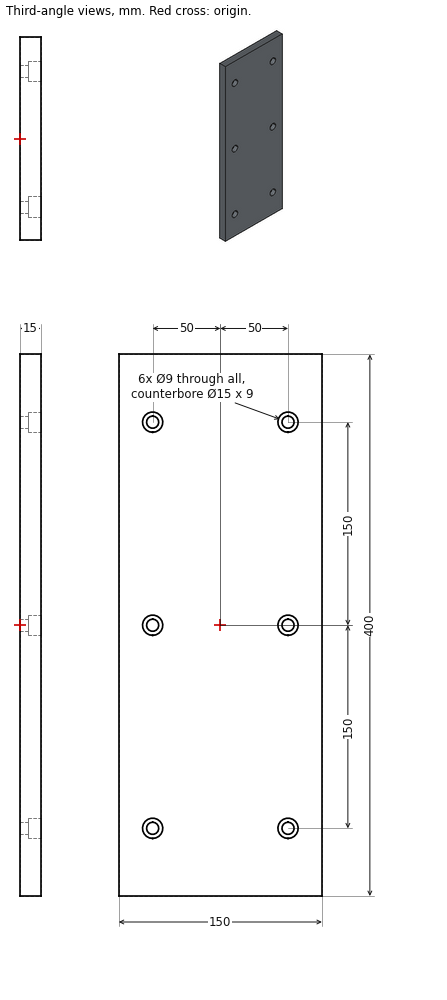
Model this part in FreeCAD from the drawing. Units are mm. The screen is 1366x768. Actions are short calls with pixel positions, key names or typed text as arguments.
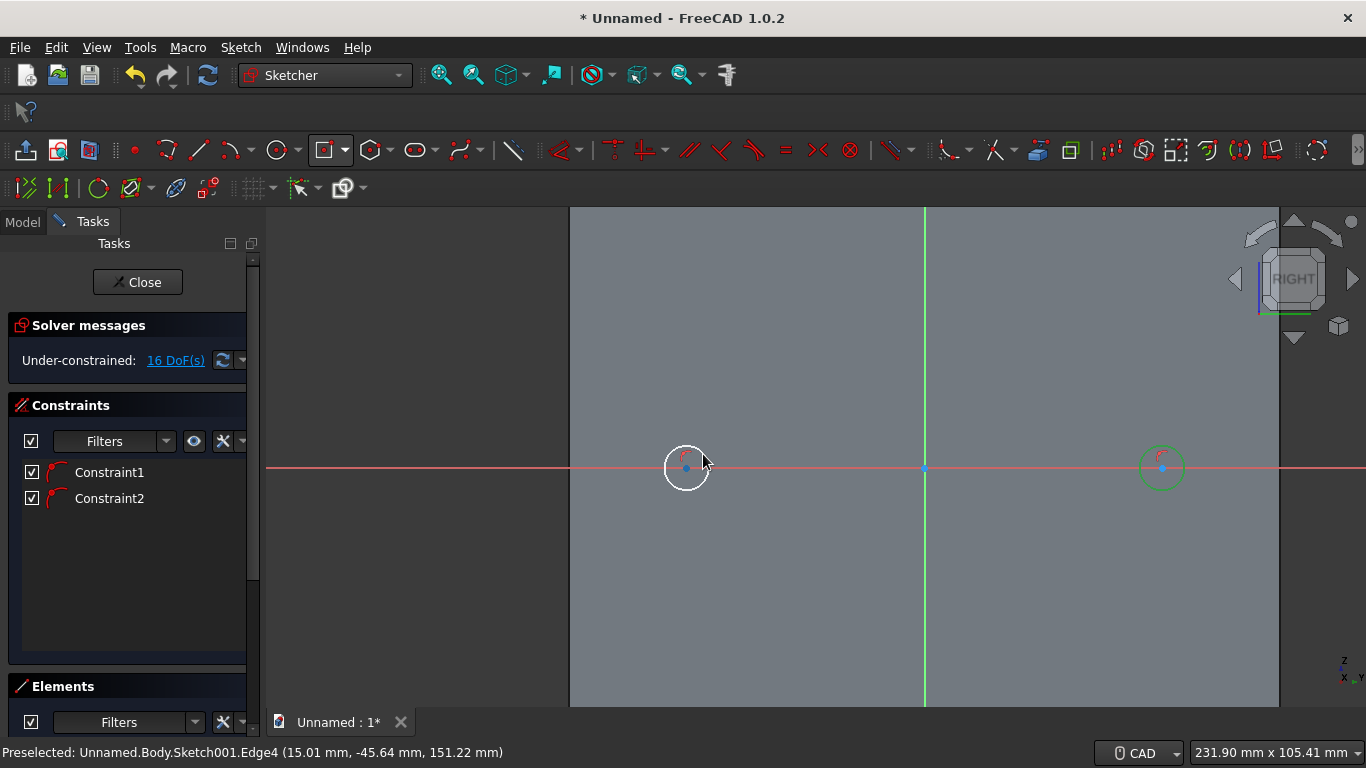
click(702, 452)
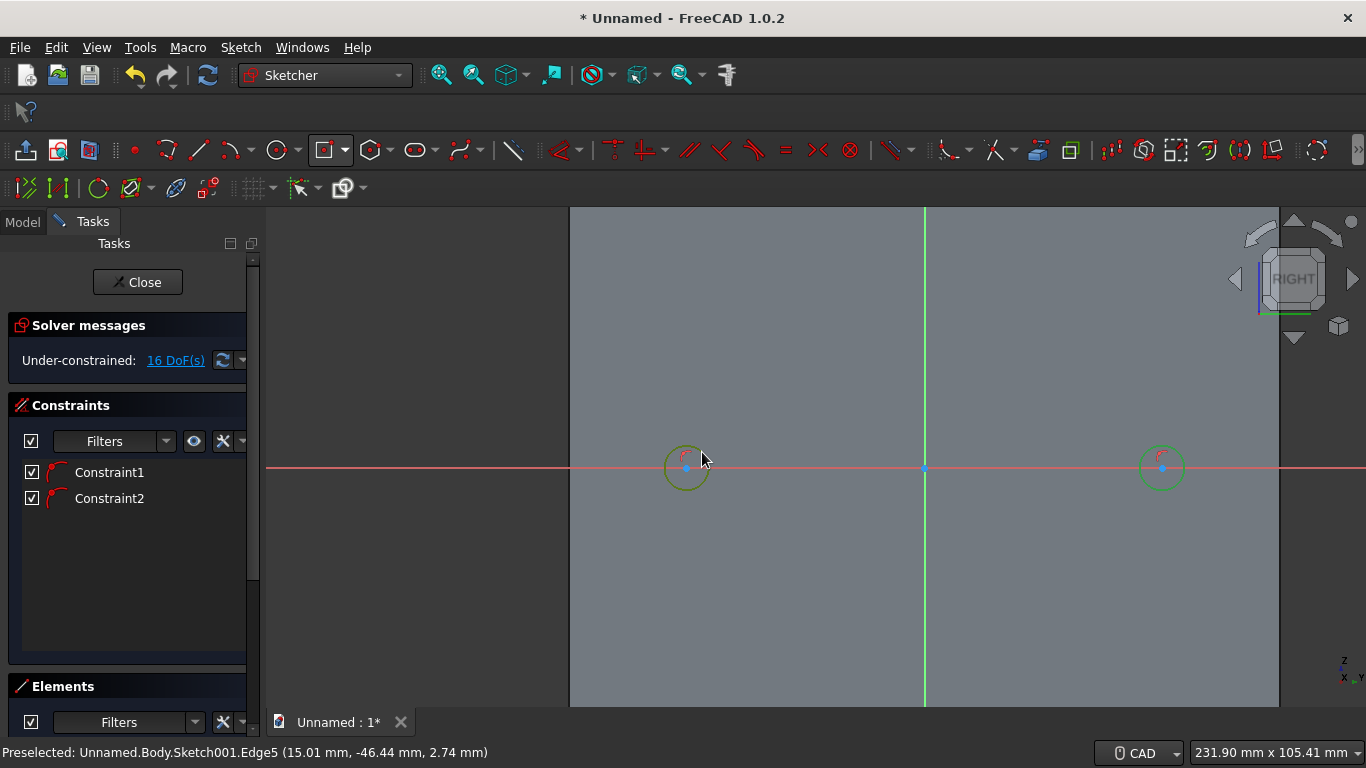
scroll(703, 454, down, 8)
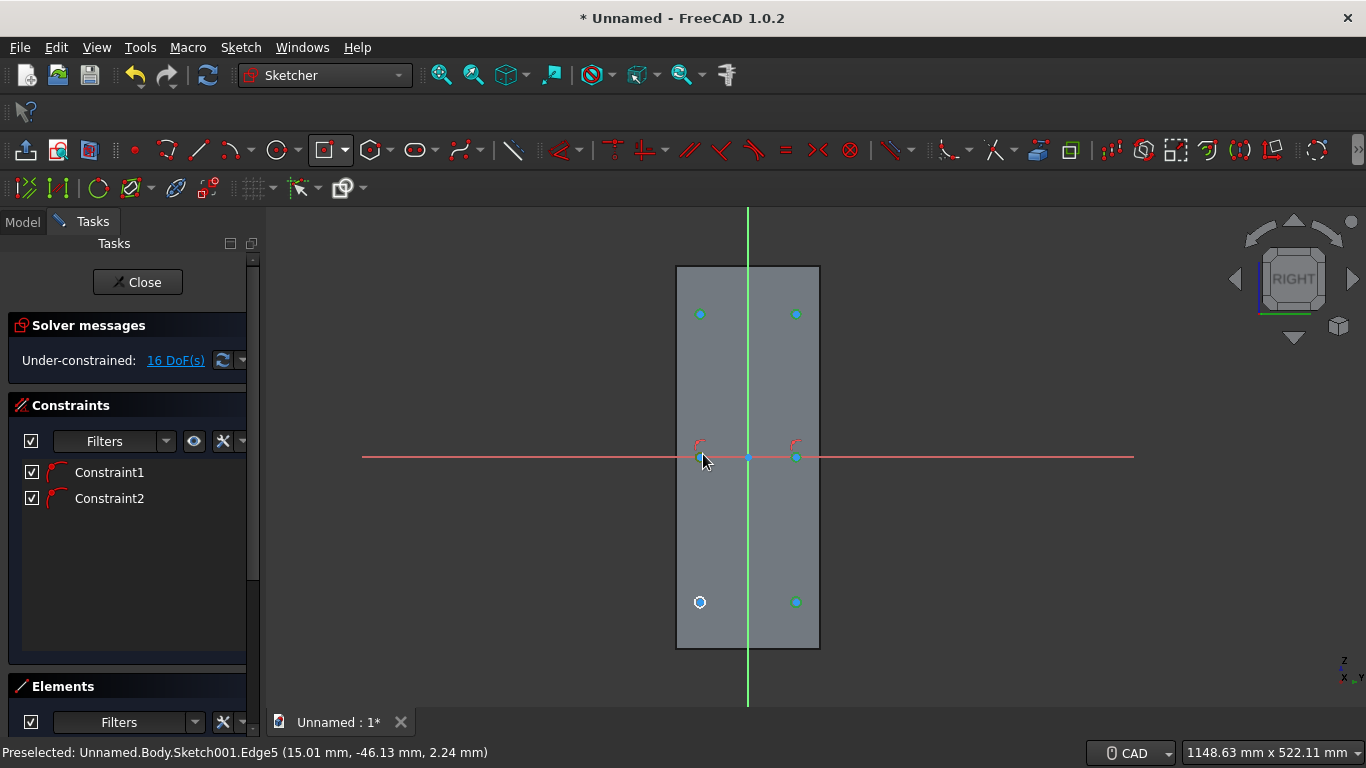
scroll(704, 599, up, 5)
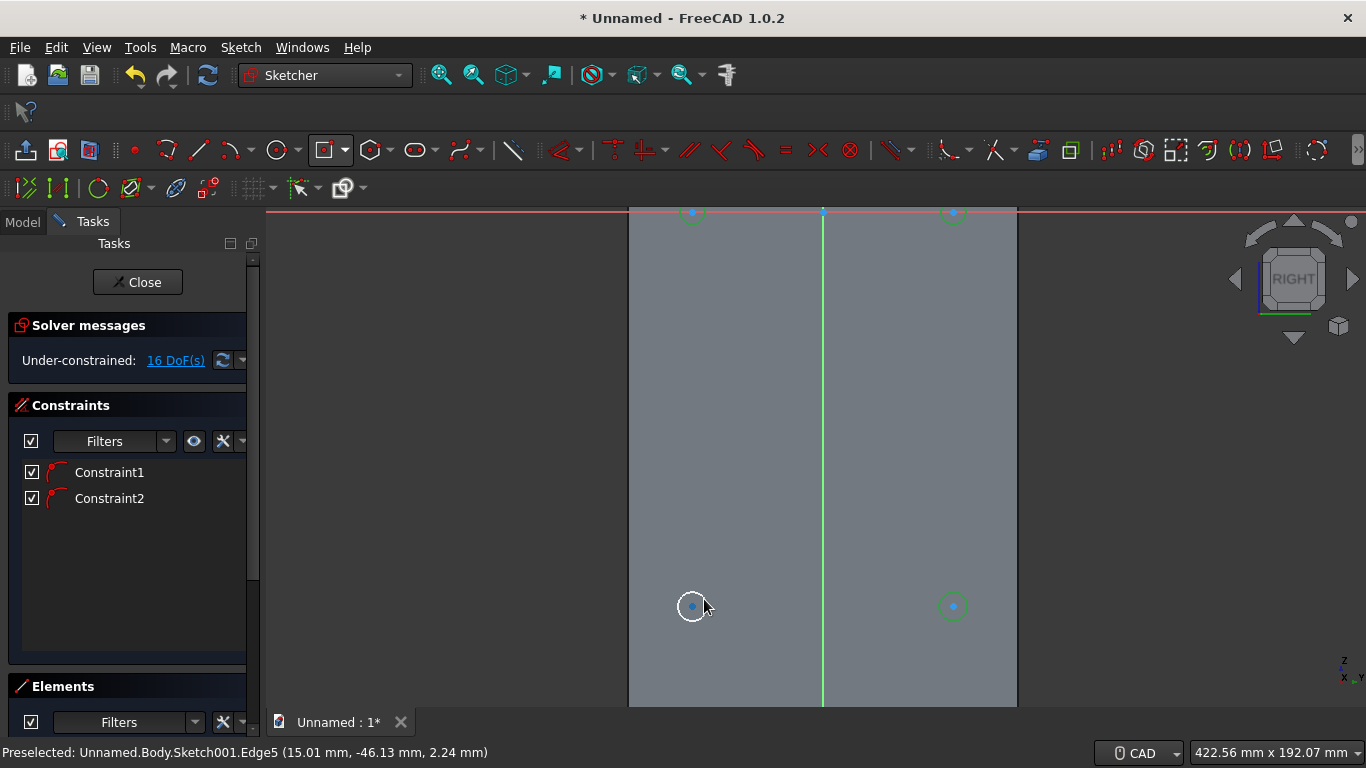
click(703, 596)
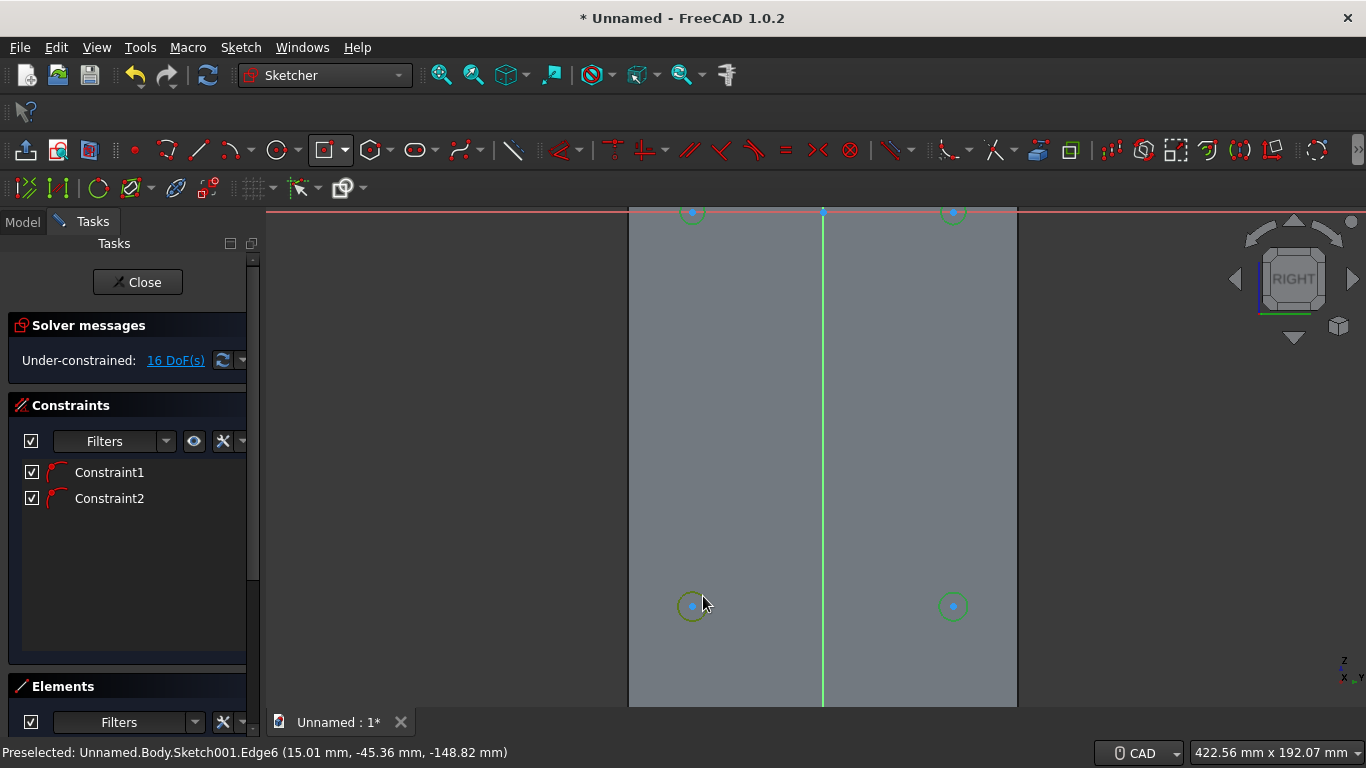
key(e)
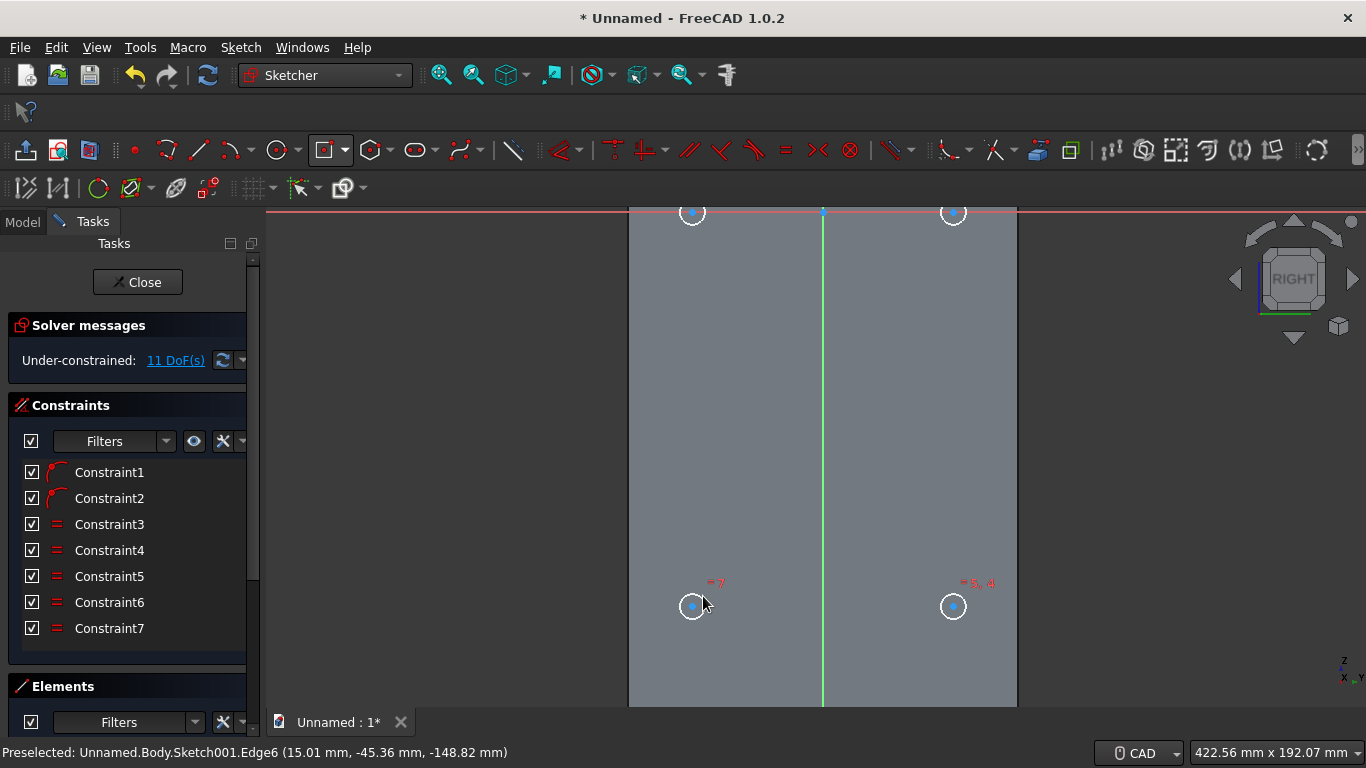
scroll(703, 599, down, 5)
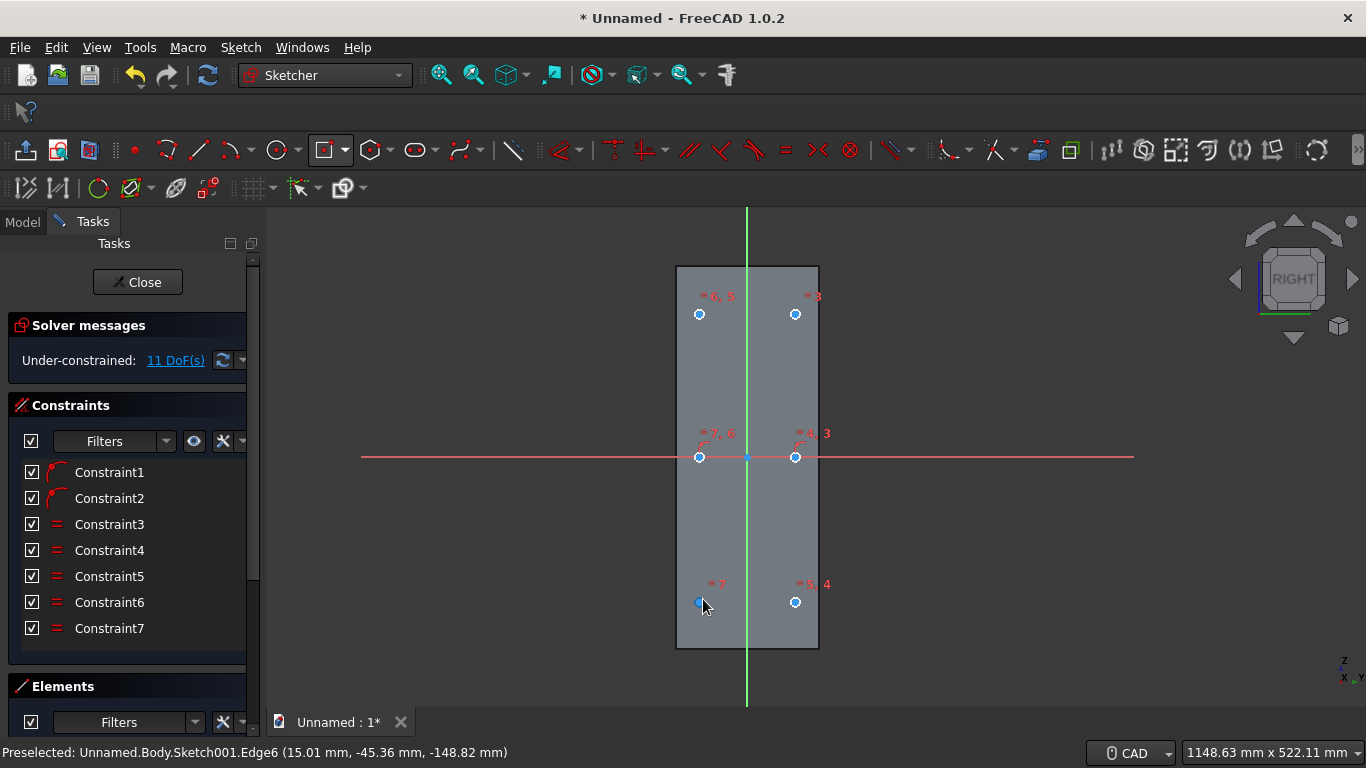
click(795, 314)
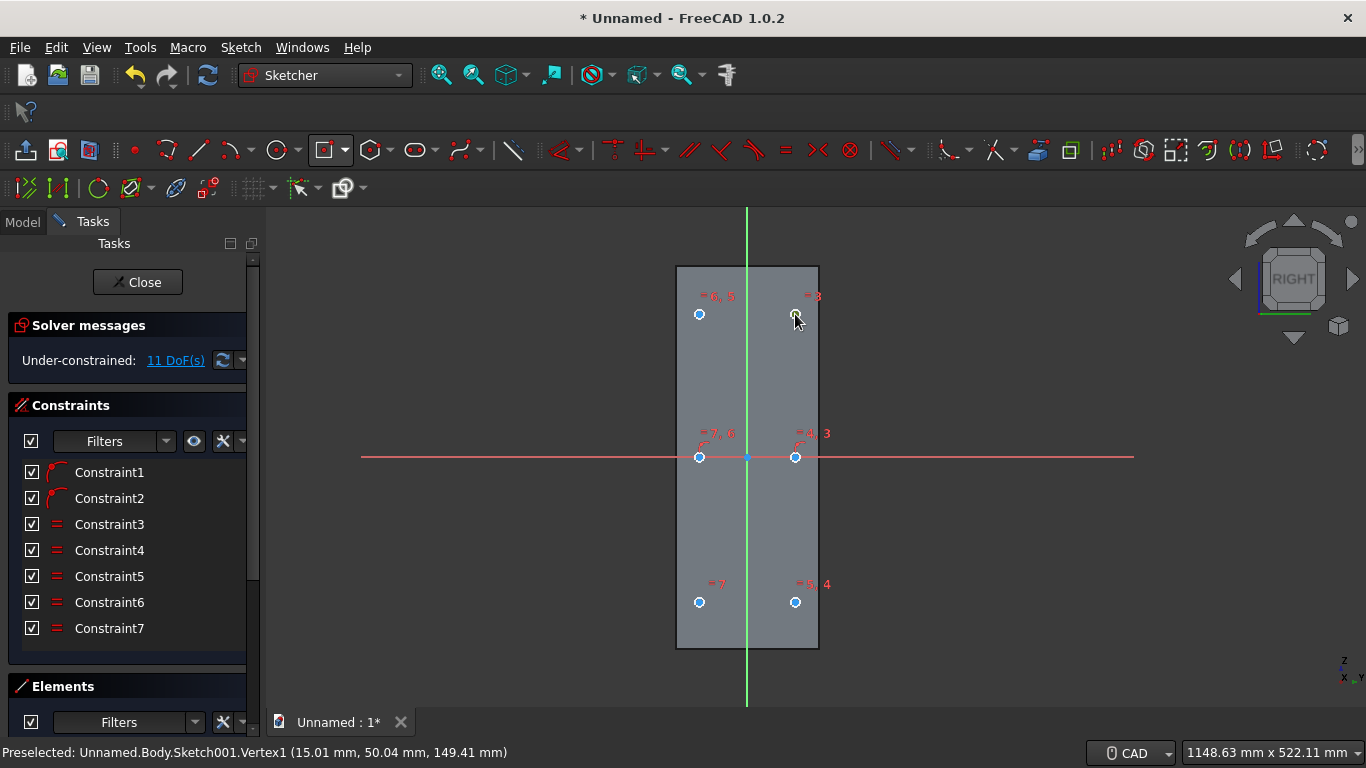
click(795, 457)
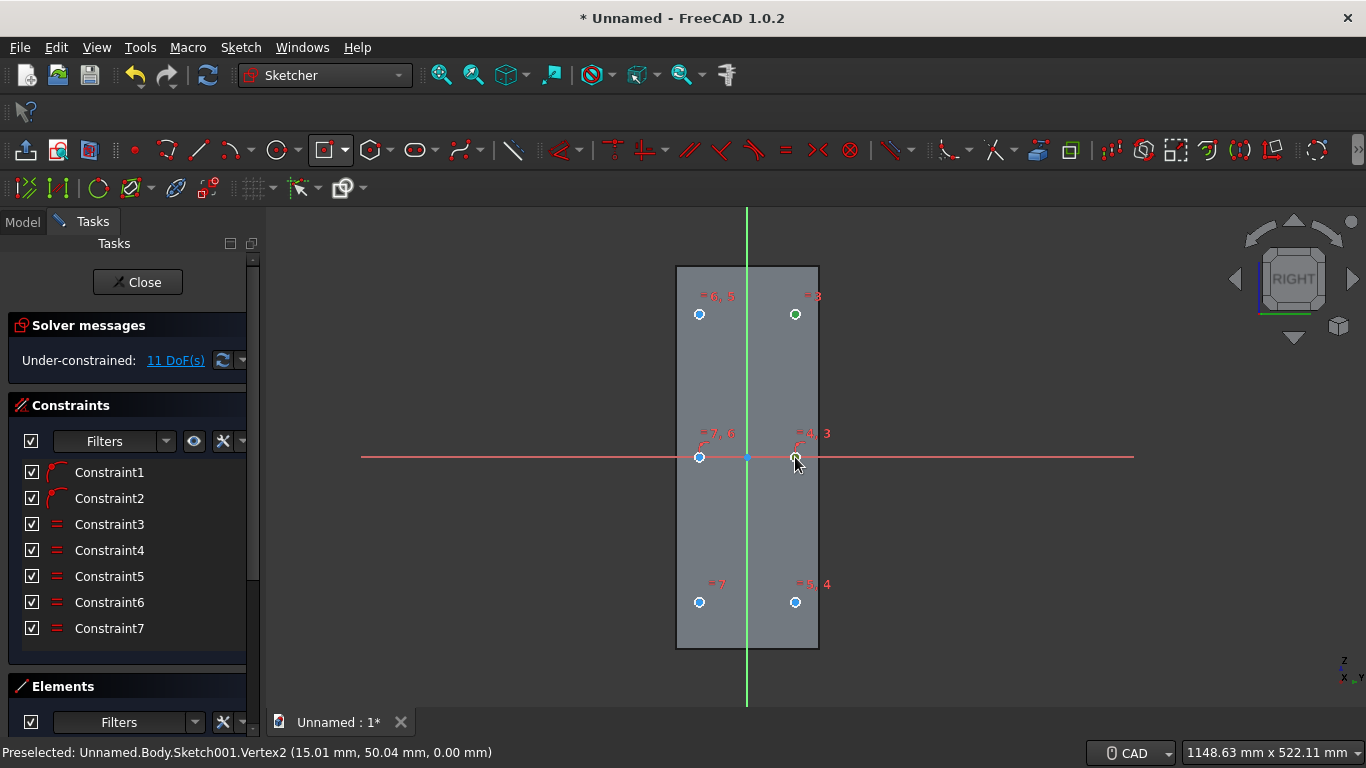
key(v)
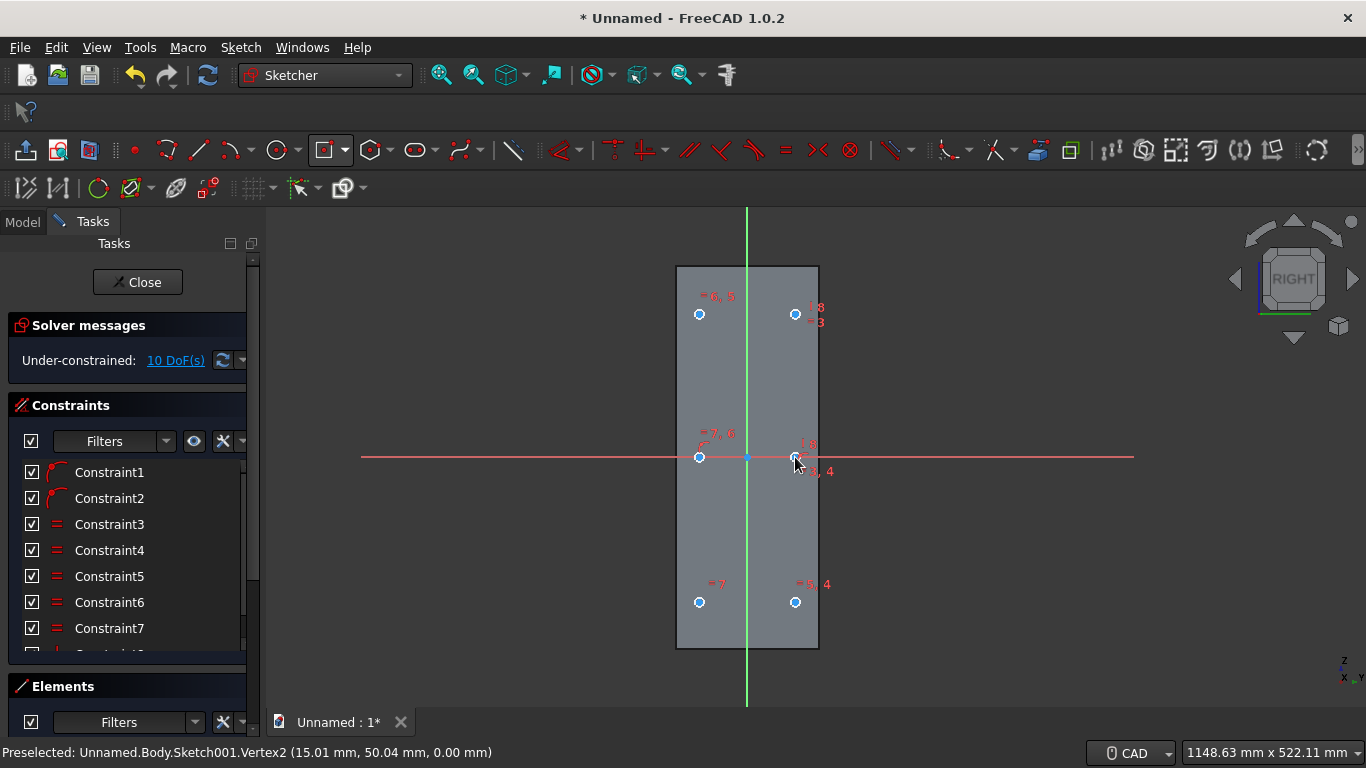
click(795, 457)